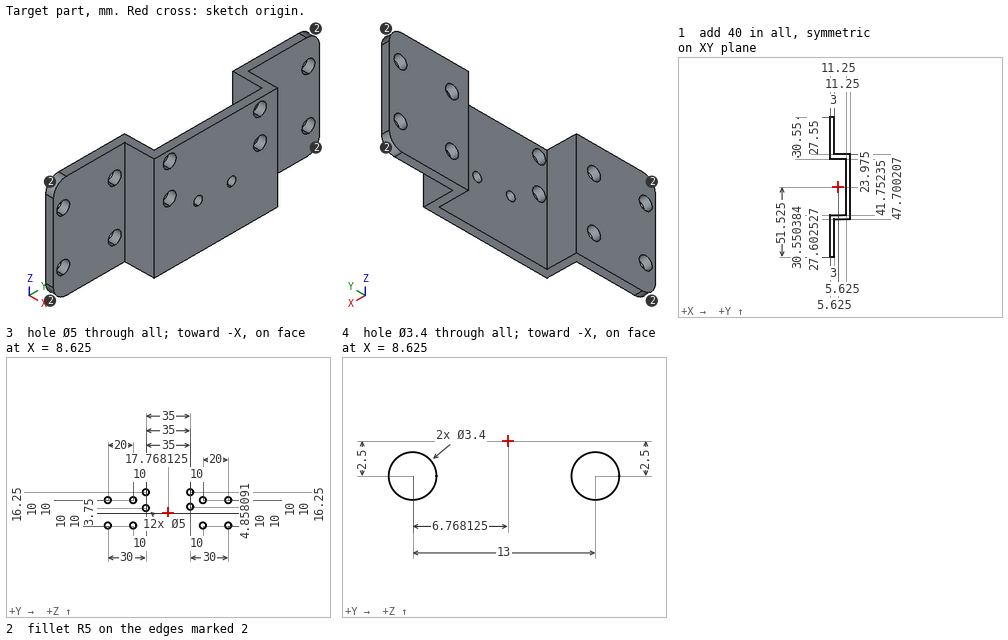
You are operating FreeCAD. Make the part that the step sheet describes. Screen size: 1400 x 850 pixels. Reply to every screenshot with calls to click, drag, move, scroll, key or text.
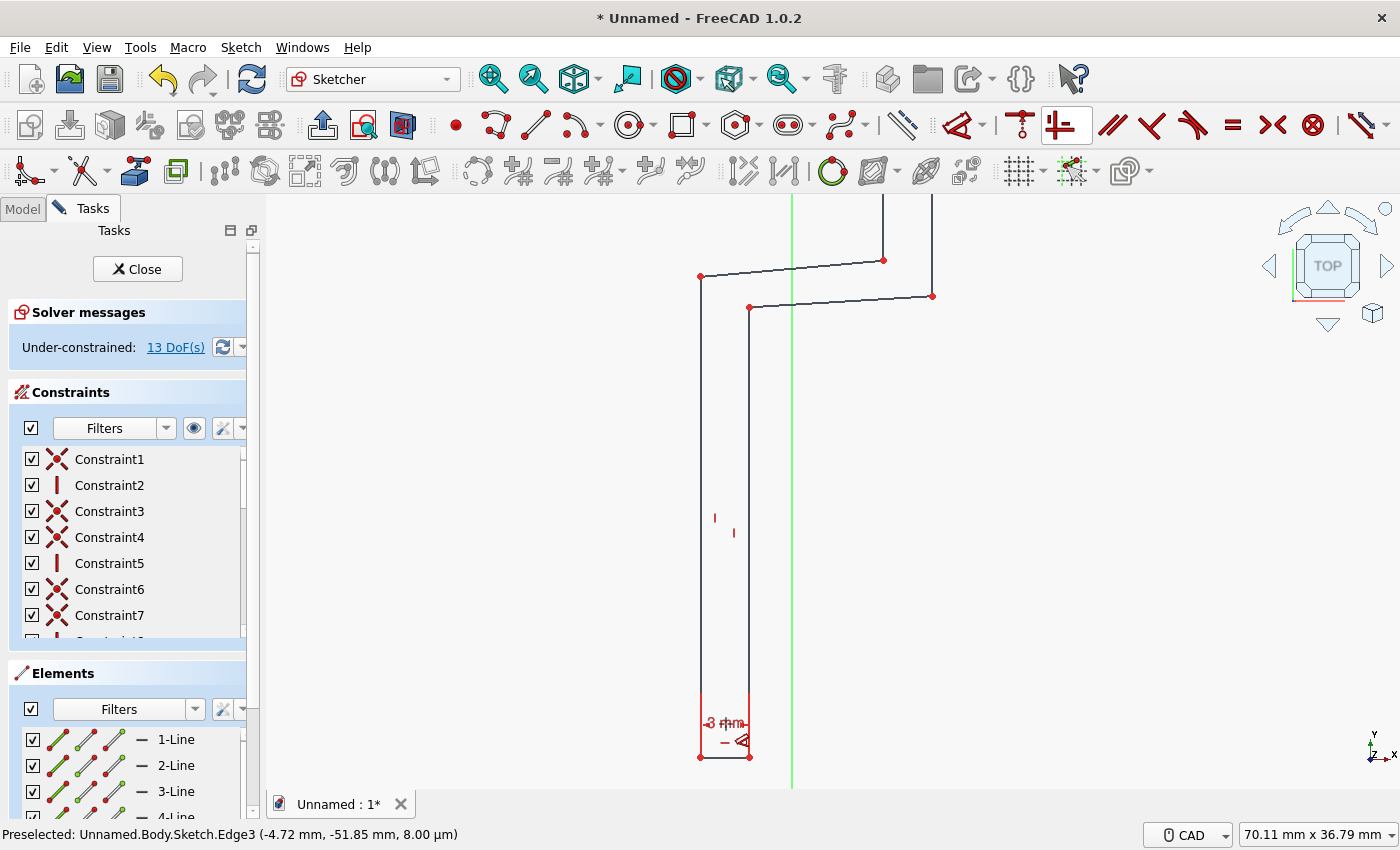
scroll(747, 679, down, 7)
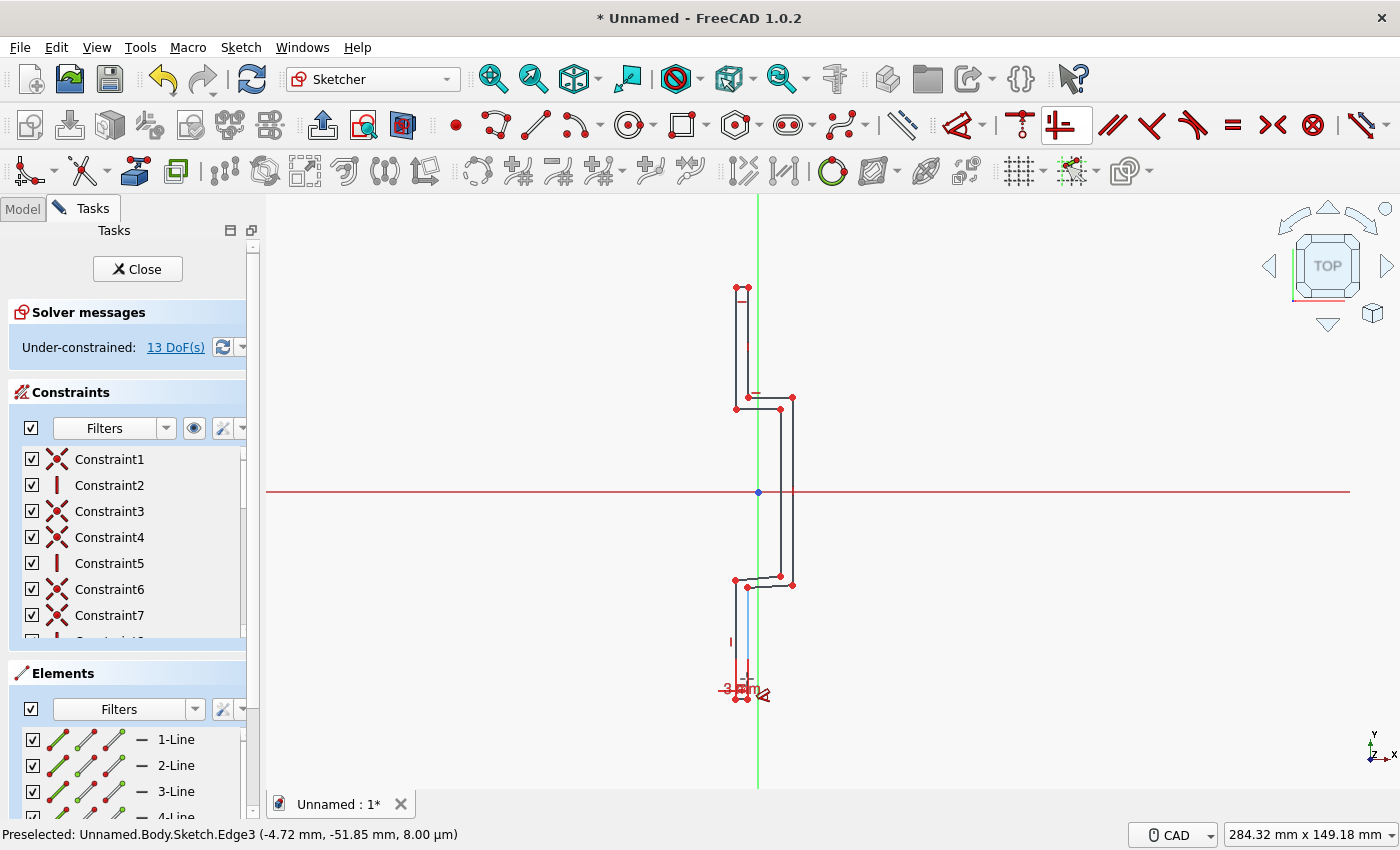
scroll(745, 287, up, 7)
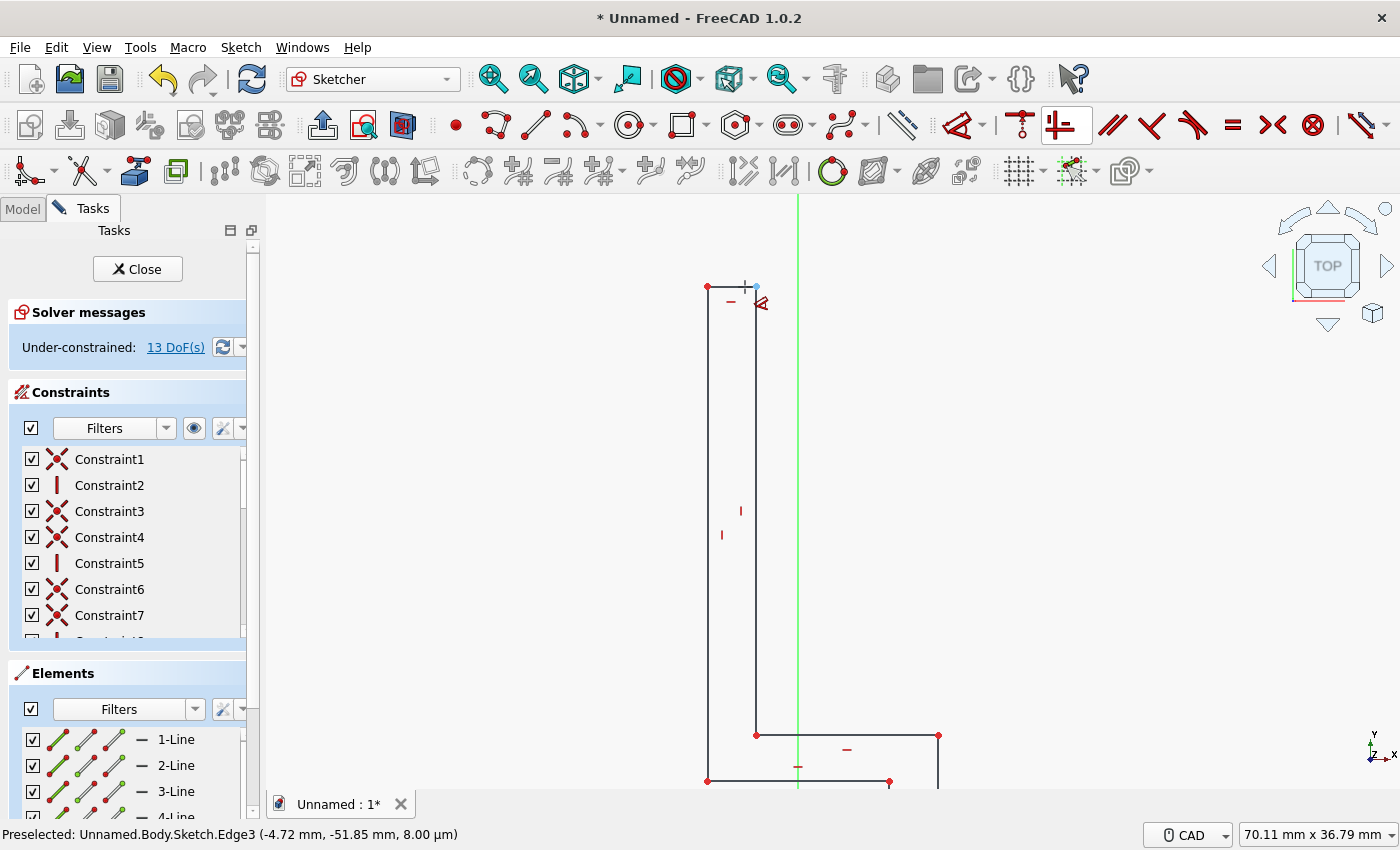
click(742, 287)
click(732, 253)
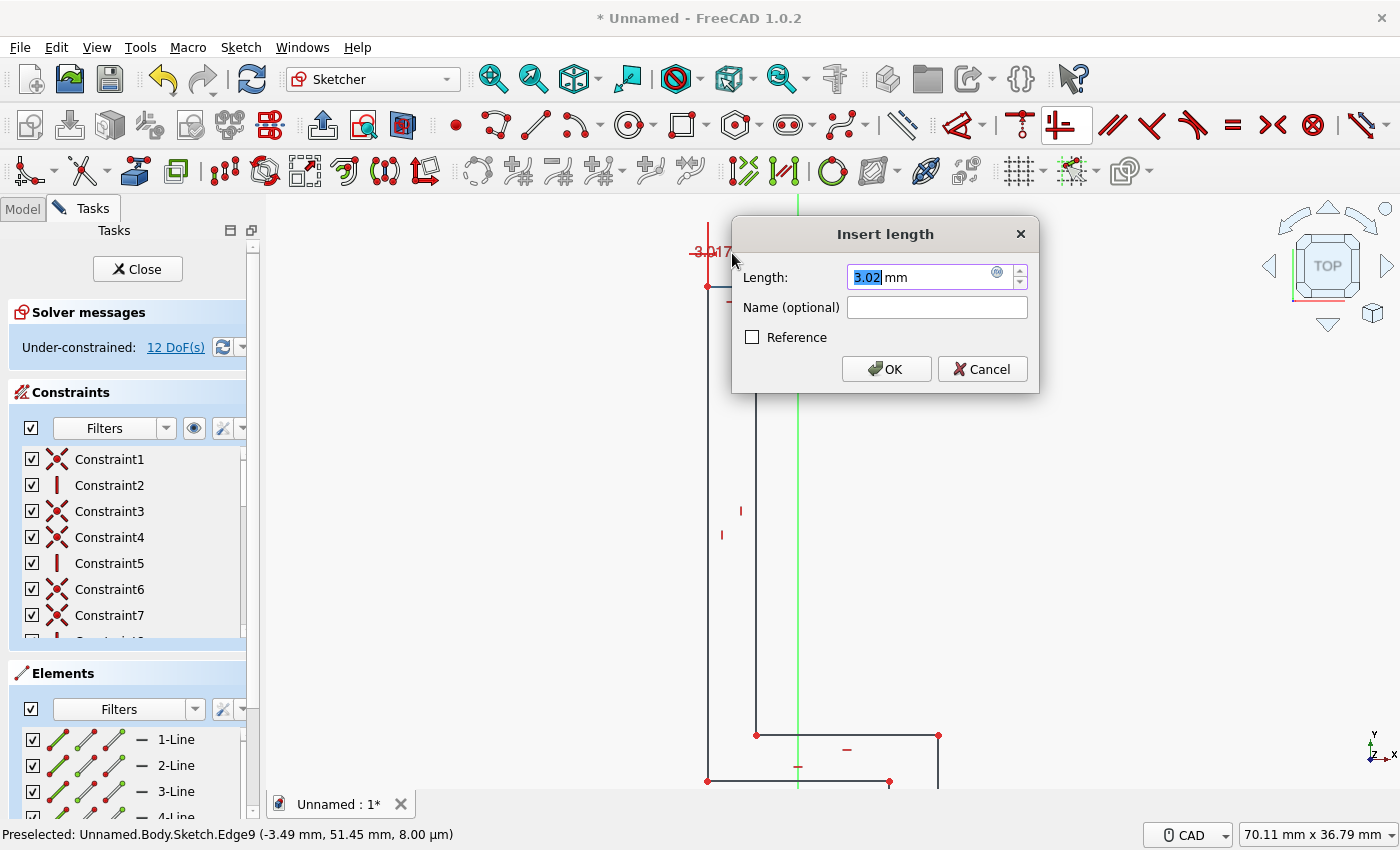
text(3)
key(Return)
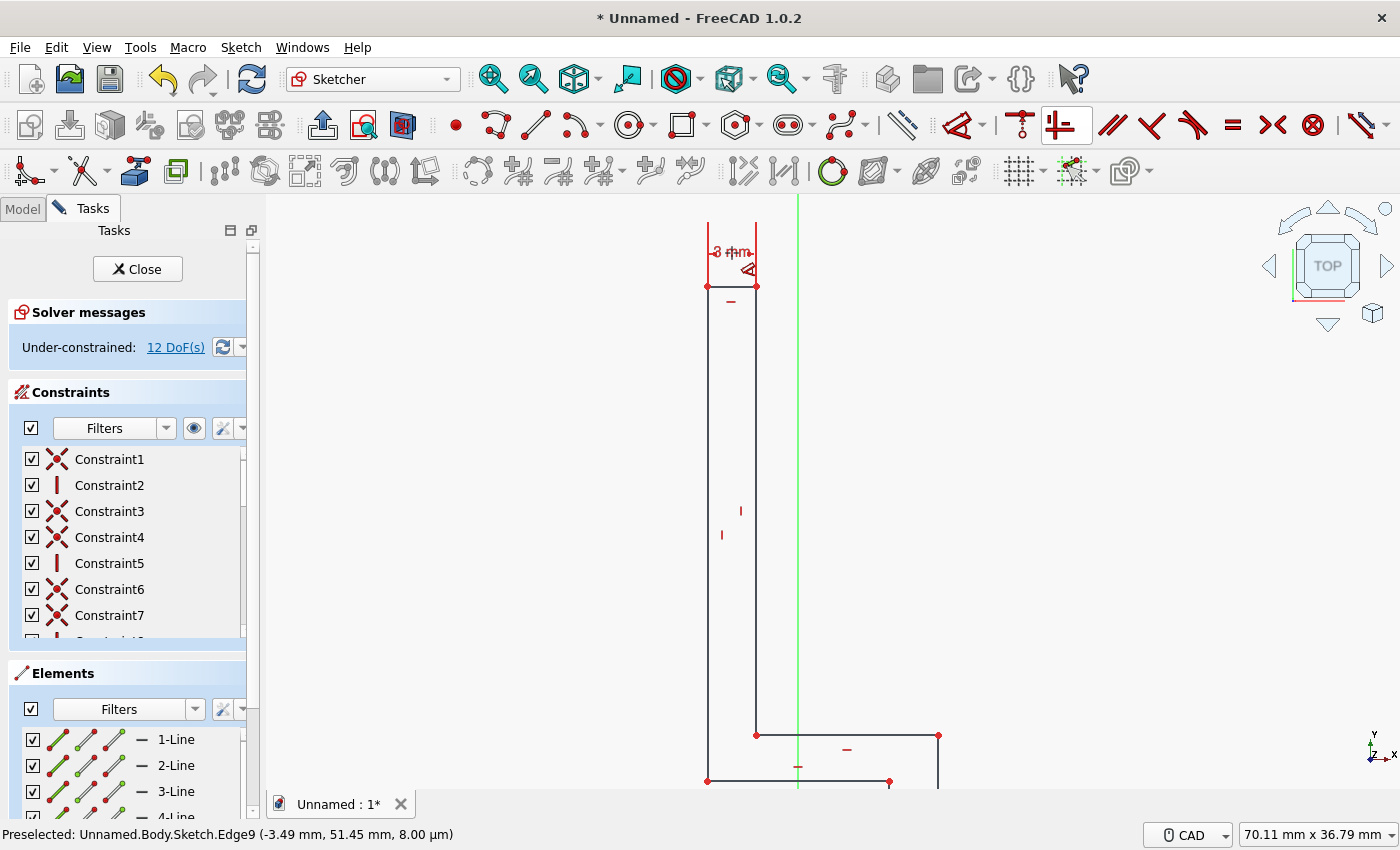
scroll(745, 286, down, 7)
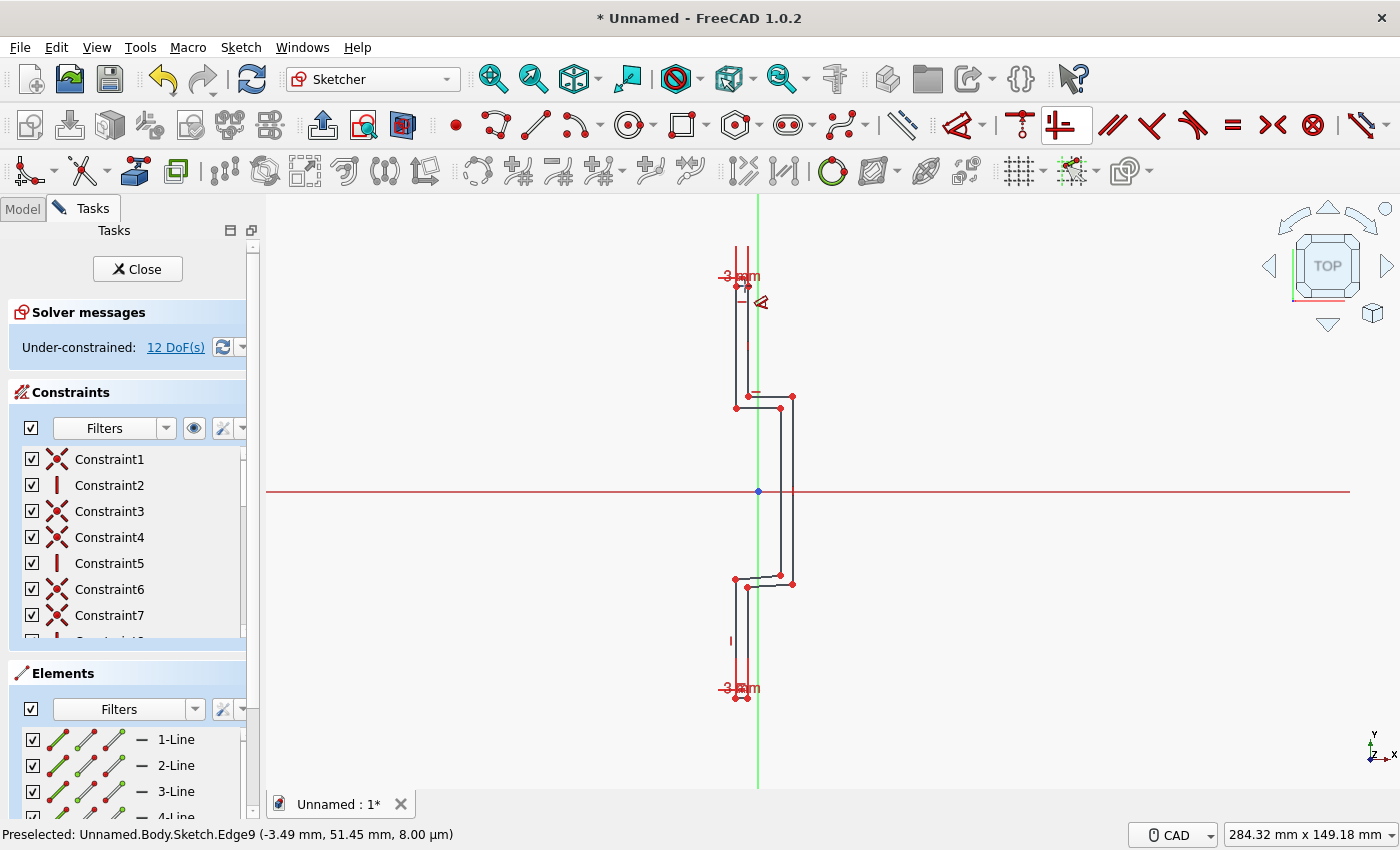
click(779, 397)
click(781, 363)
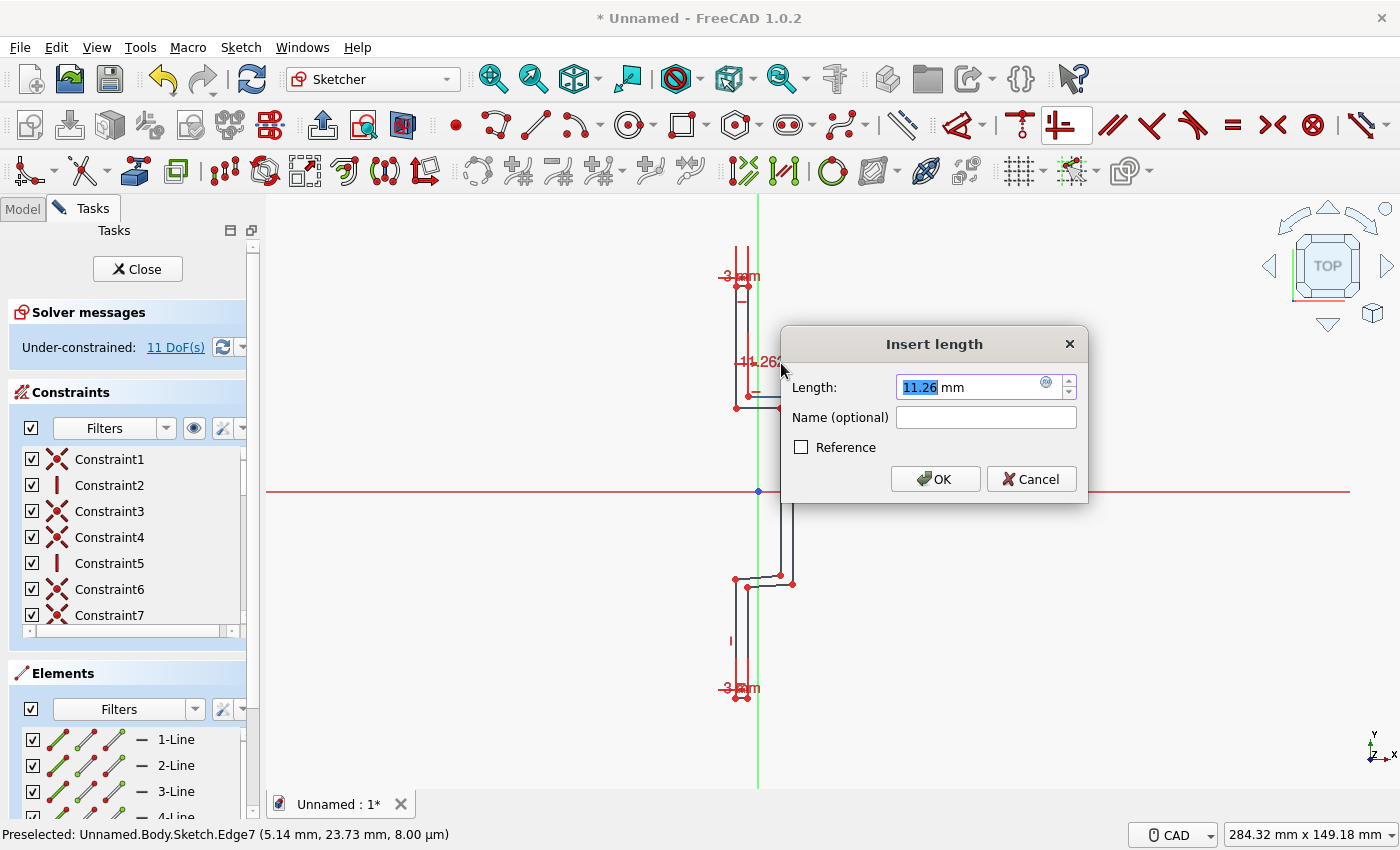
text(11.25)
key(Return)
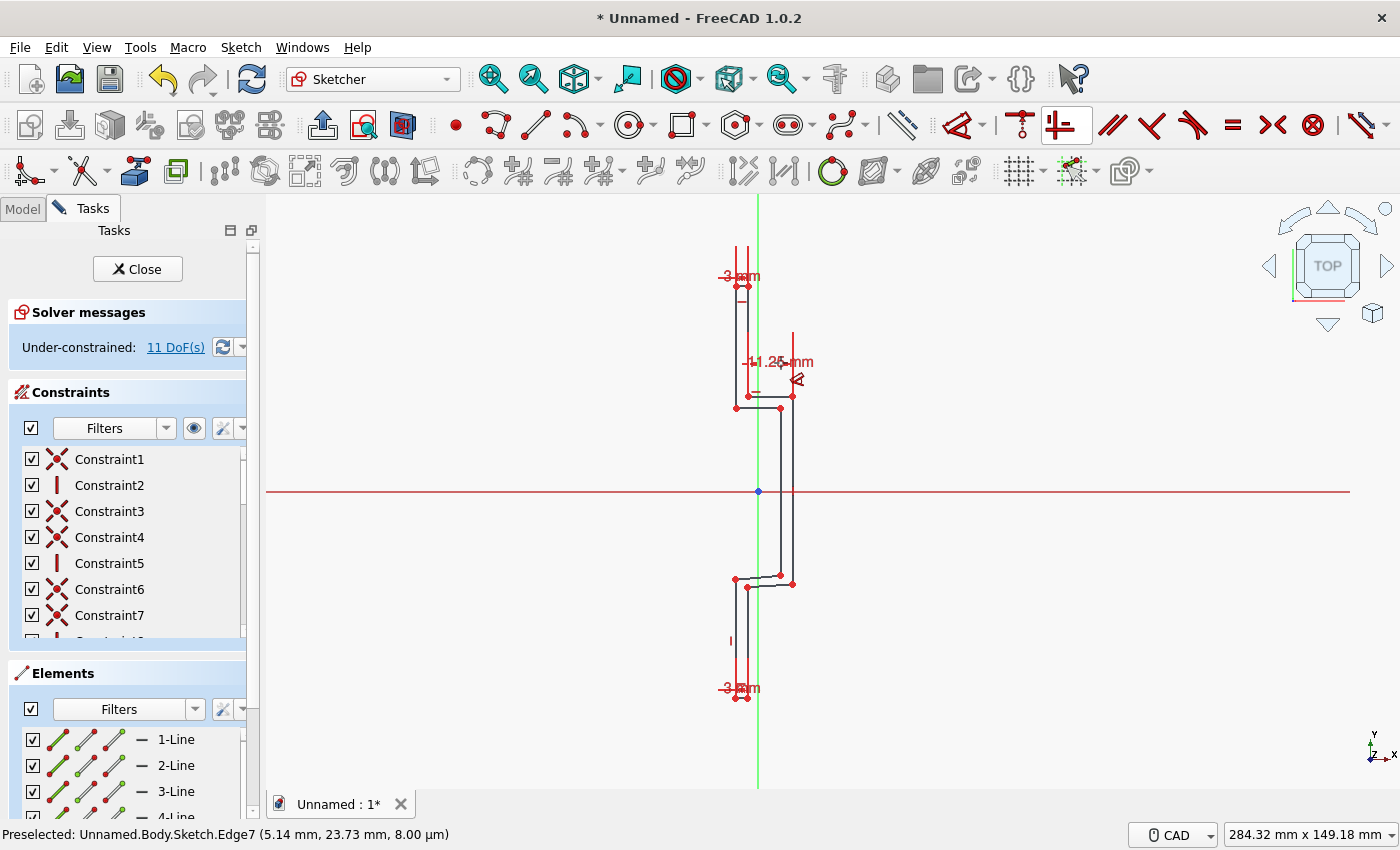
scroll(748, 364, up, 2)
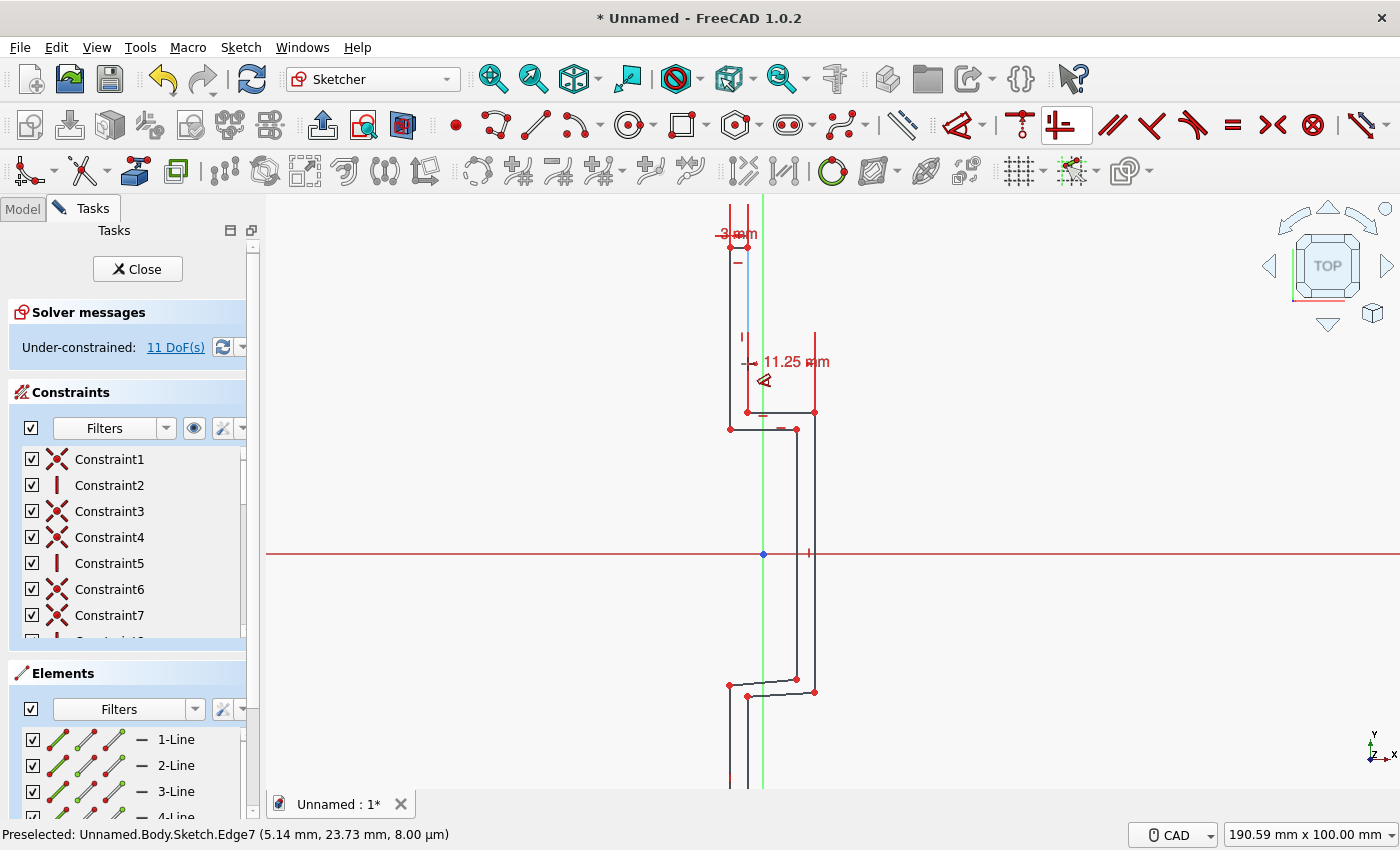
click(748, 363)
click(714, 330)